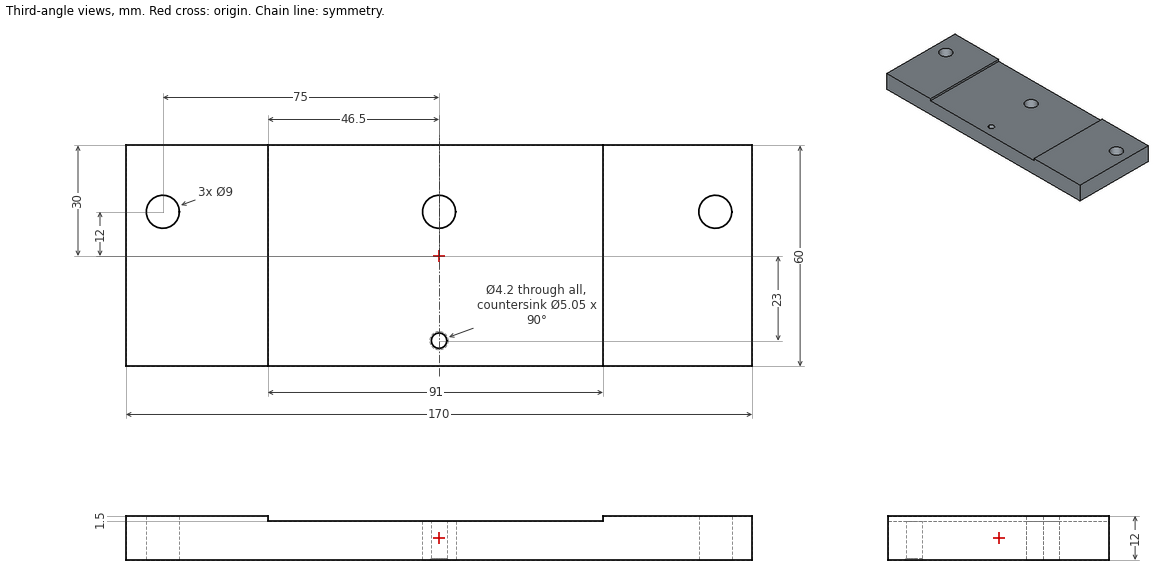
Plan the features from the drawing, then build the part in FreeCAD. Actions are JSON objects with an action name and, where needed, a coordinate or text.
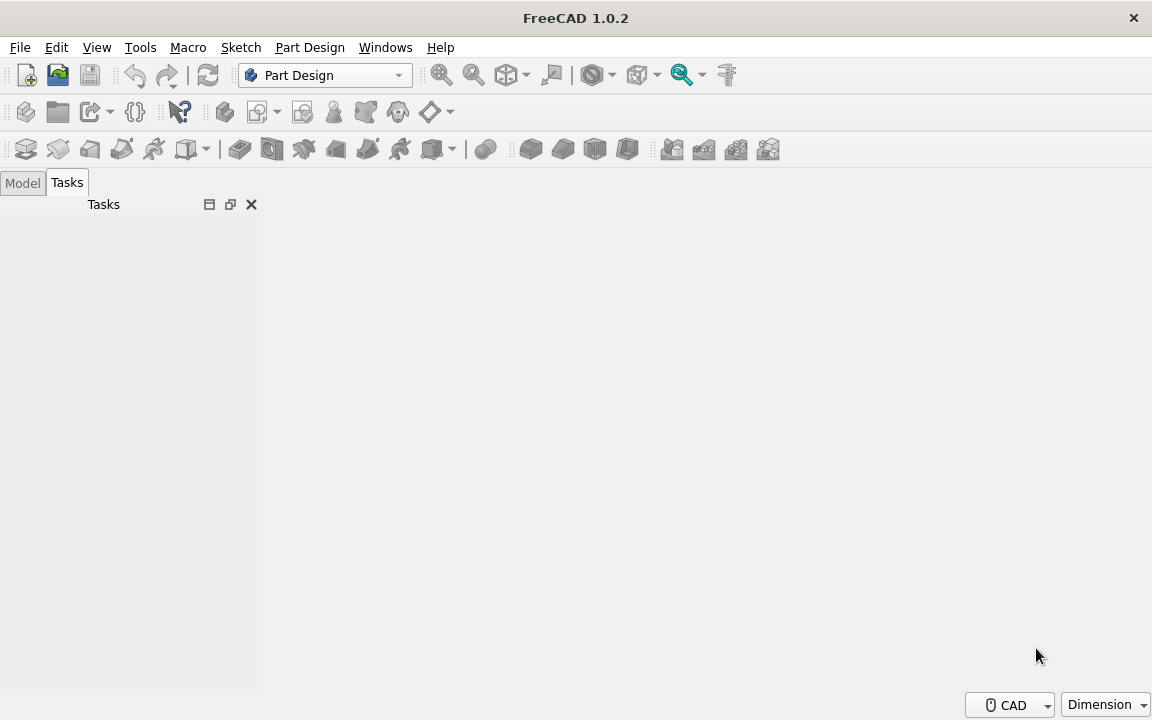
{"action": "left_click", "coordinate": [26, 76]}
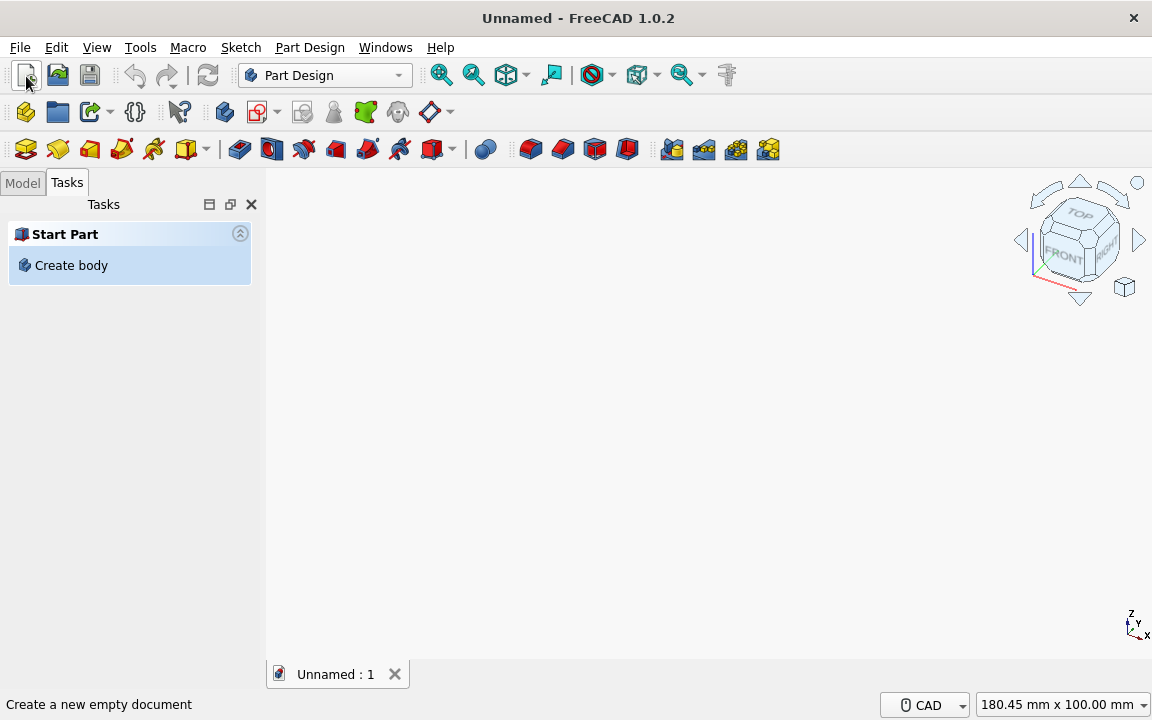
{"action": "left_click", "coordinate": [258, 112]}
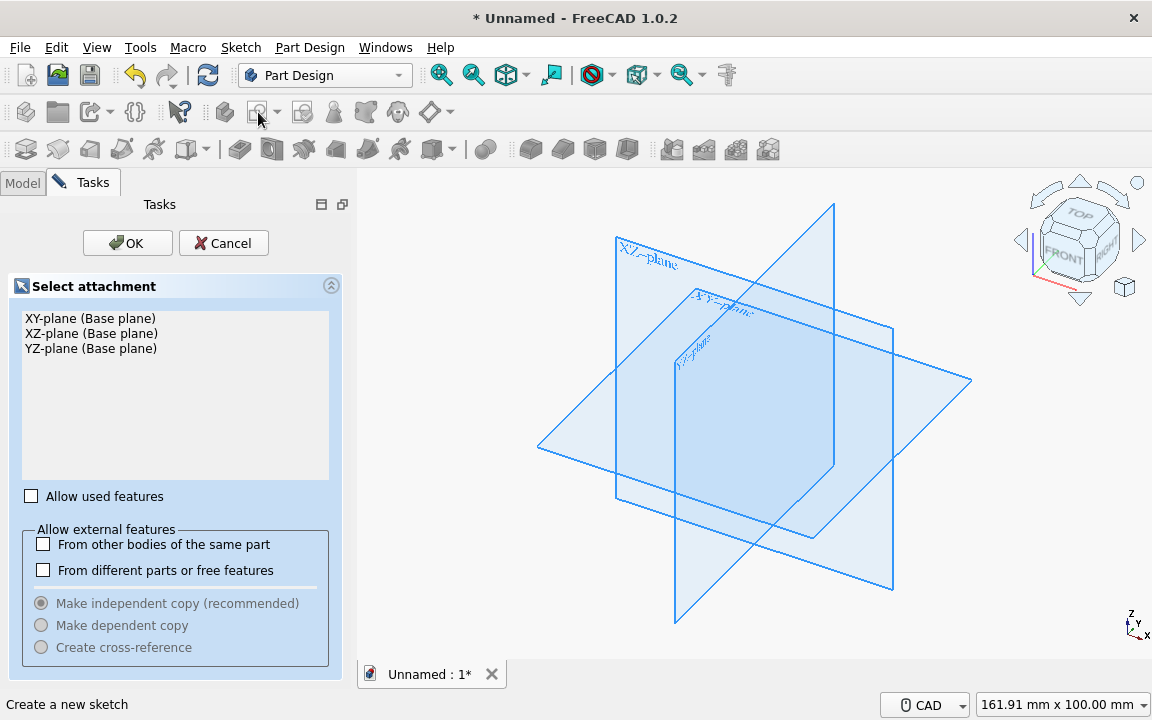
{"action": "left_click", "coordinate": [82, 318]}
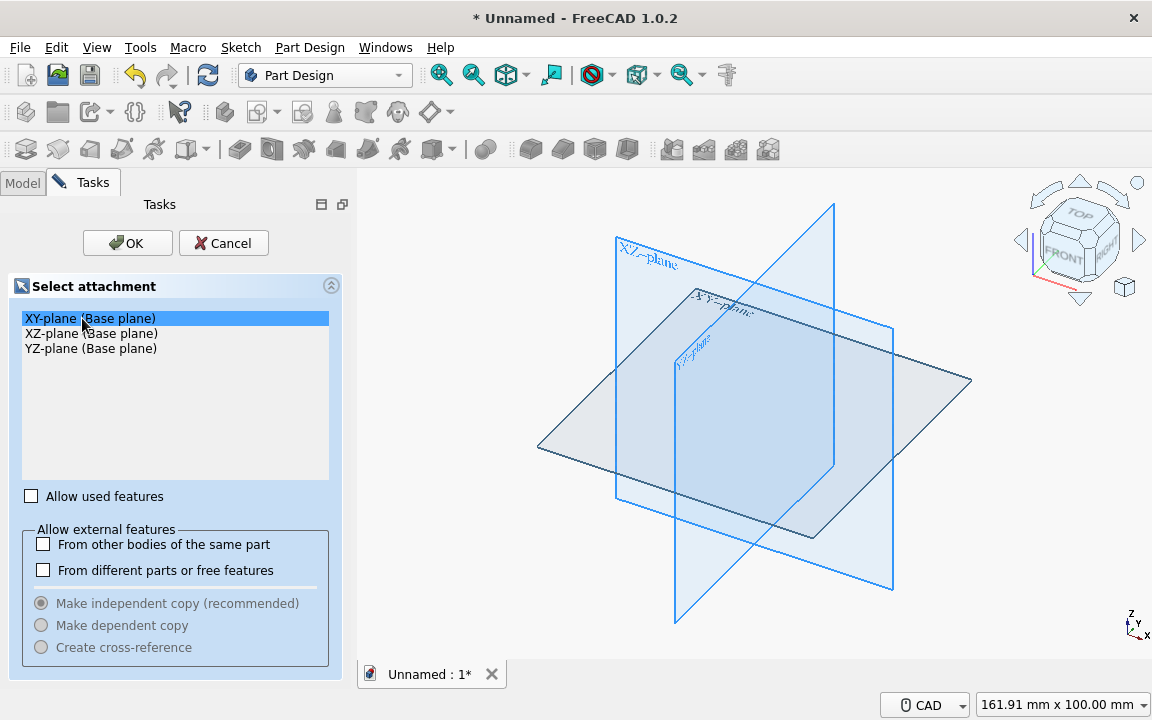
{"action": "left_click", "coordinate": [128, 243]}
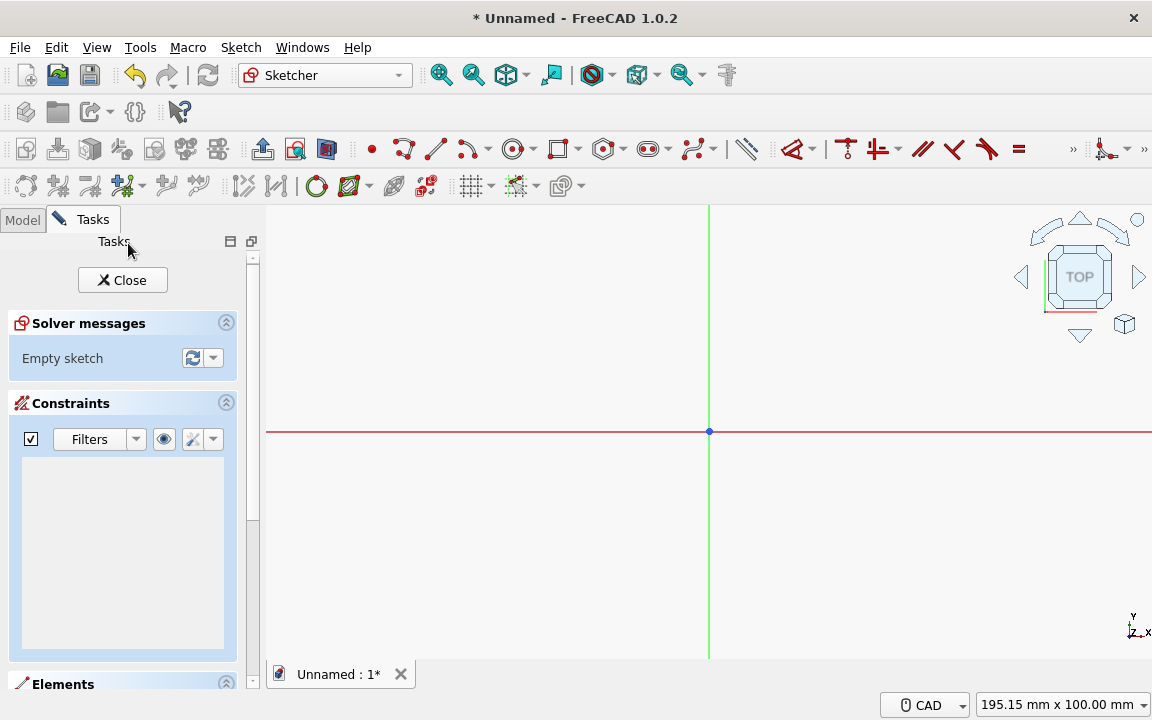
{"action": "scroll", "coordinate": [501, 432], "scroll_direction": "down", "scroll_amount": 2}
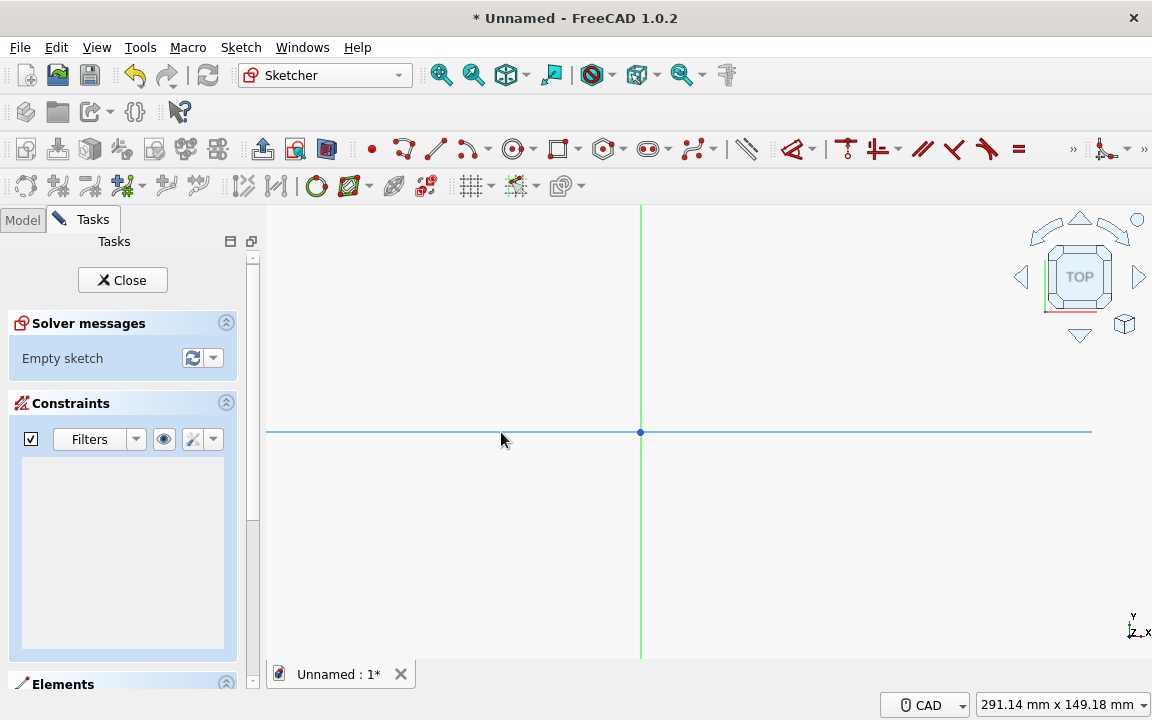
{"action": "key", "text": "g v"}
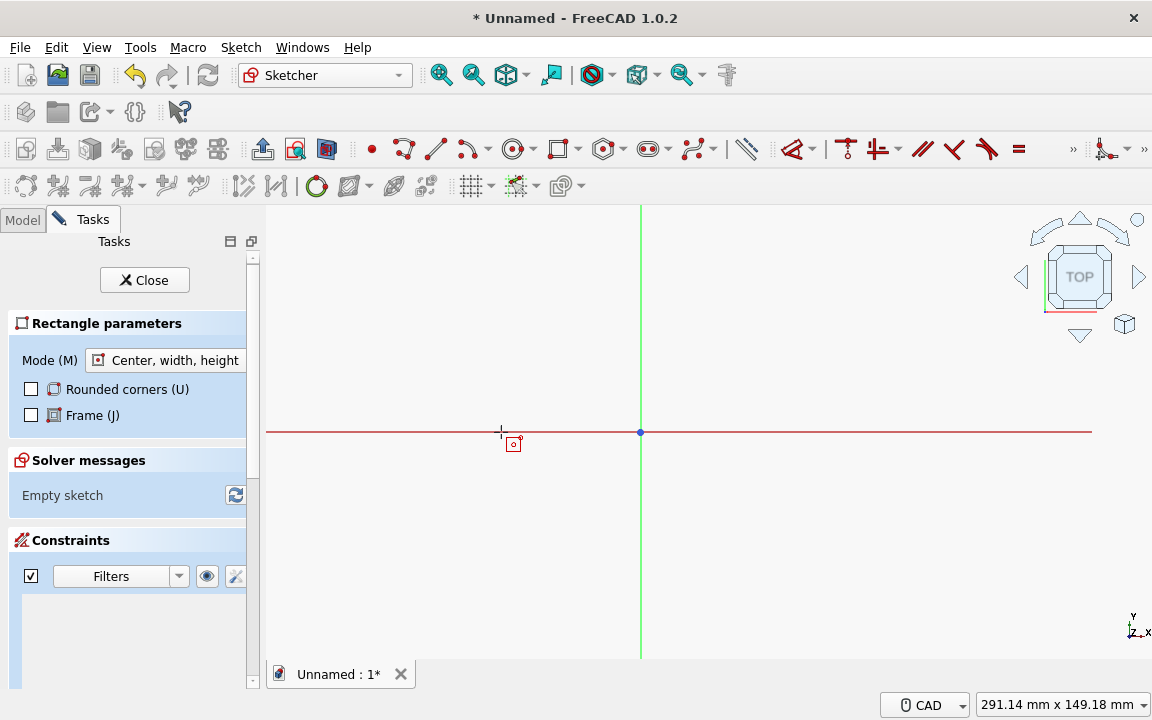
{"action": "left_click", "coordinate": [641, 432]}
{"action": "left_click", "coordinate": [899, 341]}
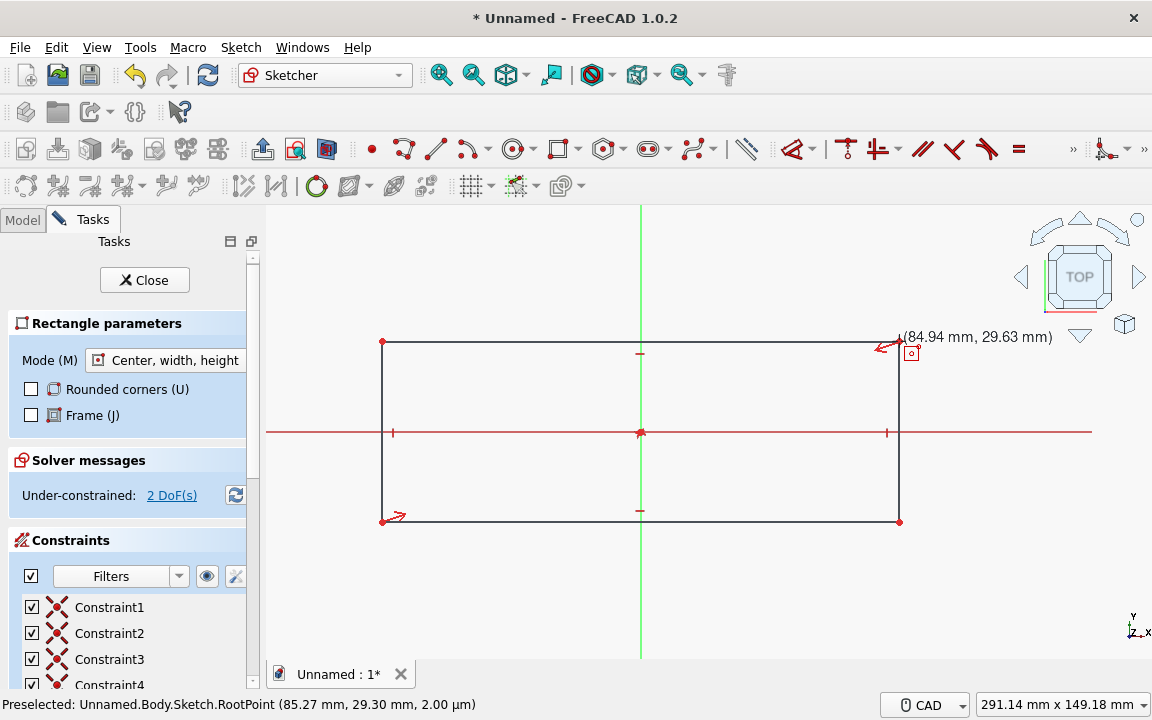
{"action": "key", "text": "g c"}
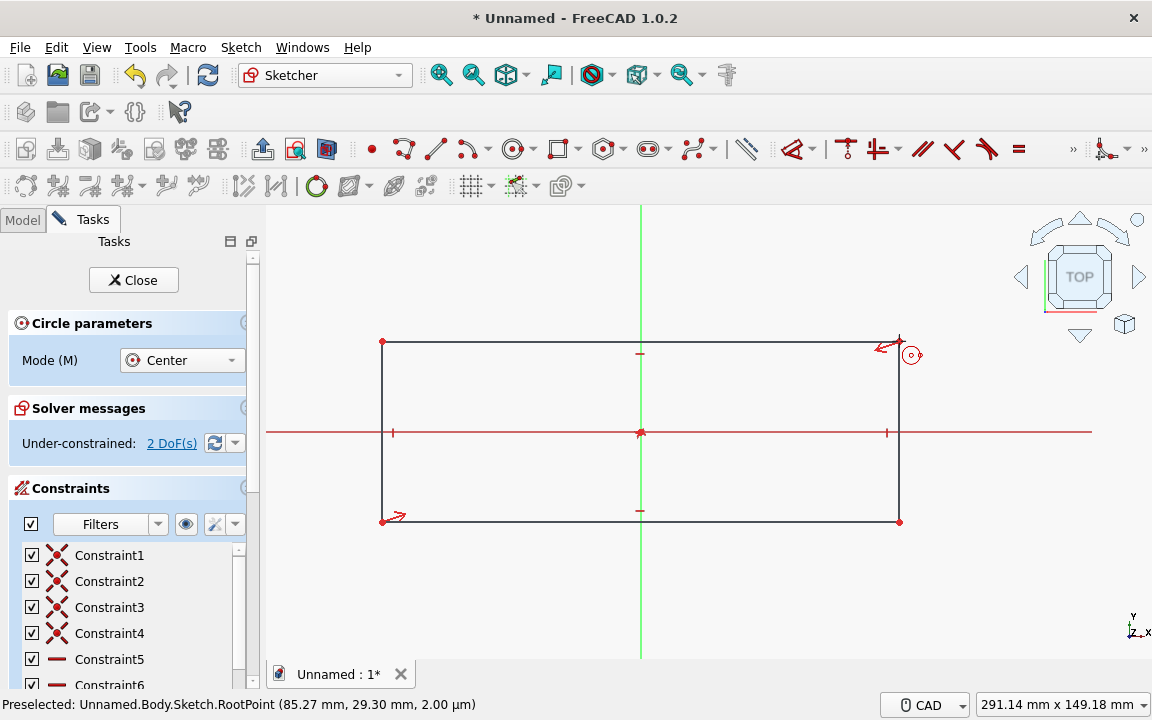
{"action": "scroll", "coordinate": [412, 396], "scroll_direction": "up", "scroll_amount": 3}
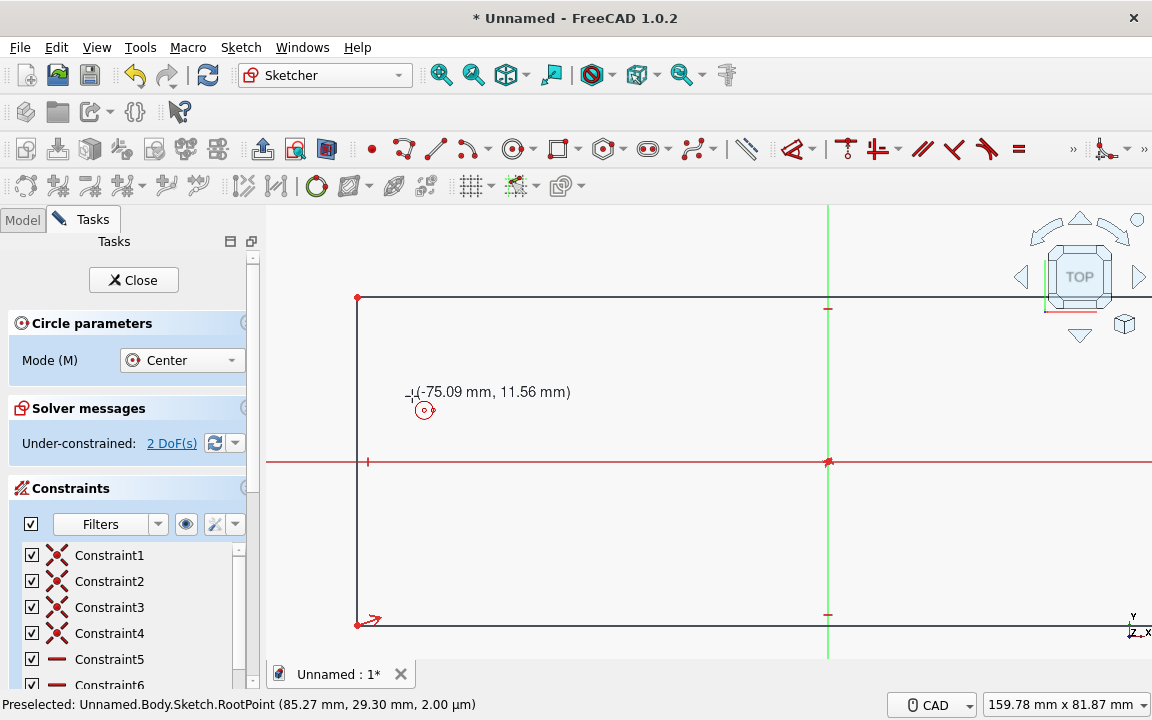
{"action": "left_click", "coordinate": [412, 395]}
{"action": "left_click", "coordinate": [430, 377]}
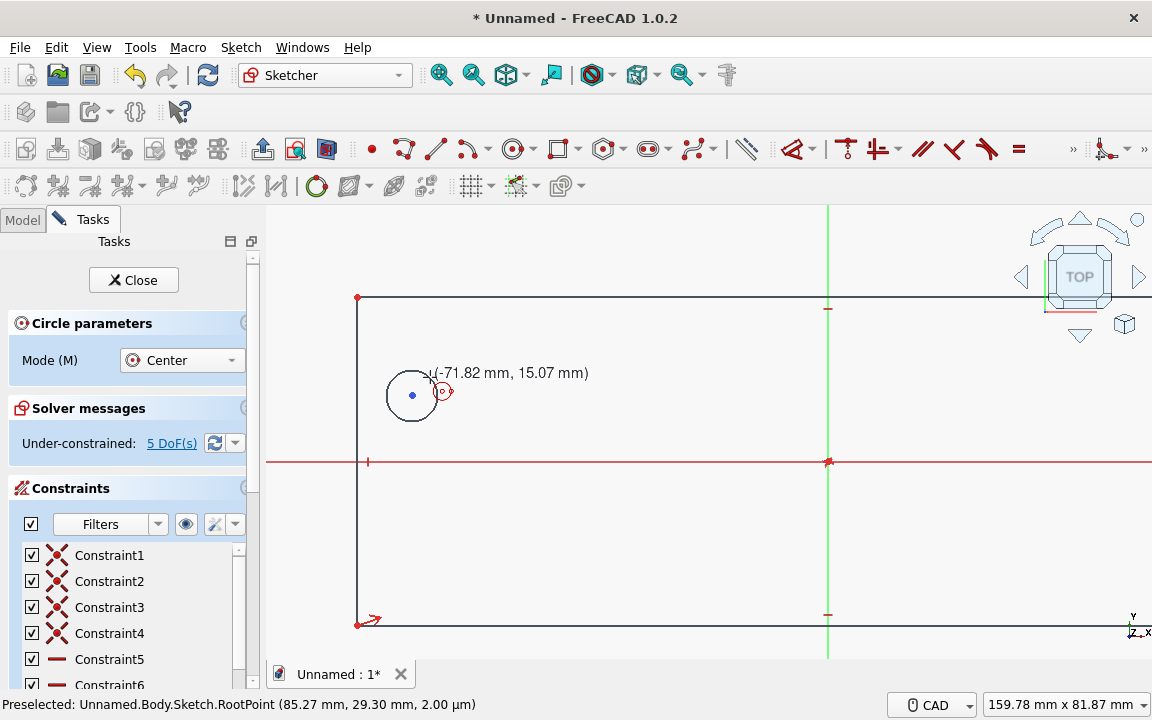
{"action": "left_click", "coordinate": [828, 395]}
{"action": "left_click", "coordinate": [846, 377]}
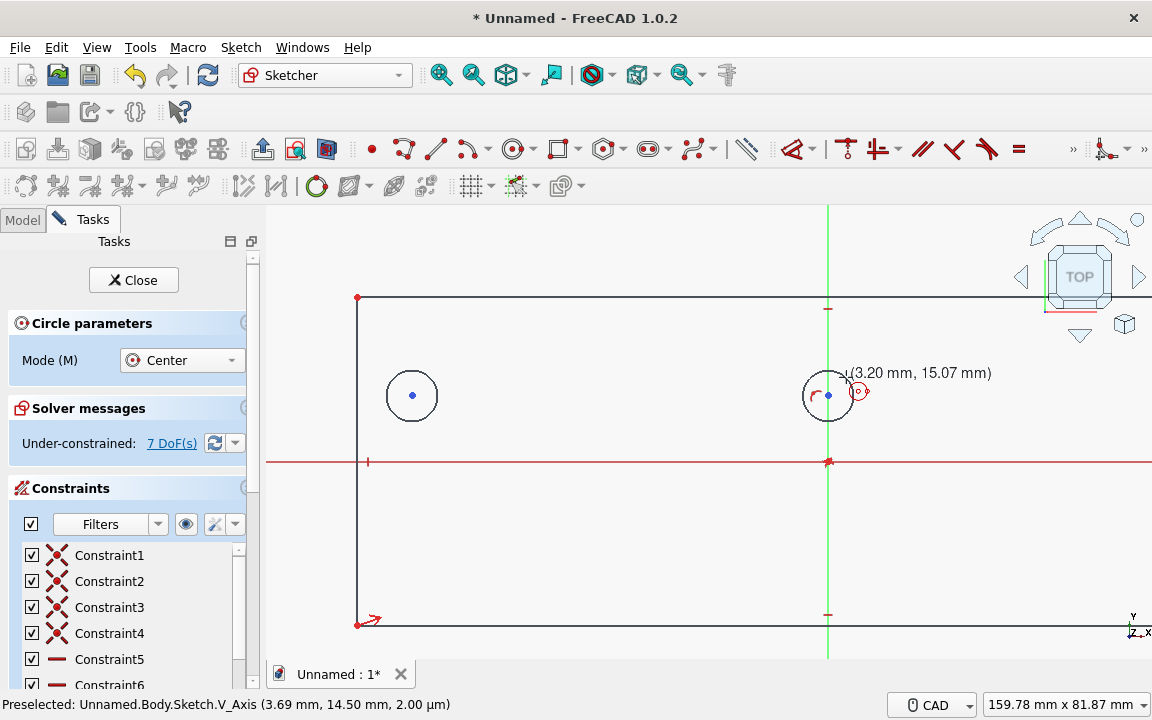
{"action": "scroll", "coordinate": [412, 396], "scroll_direction": "down", "scroll_amount": 3}